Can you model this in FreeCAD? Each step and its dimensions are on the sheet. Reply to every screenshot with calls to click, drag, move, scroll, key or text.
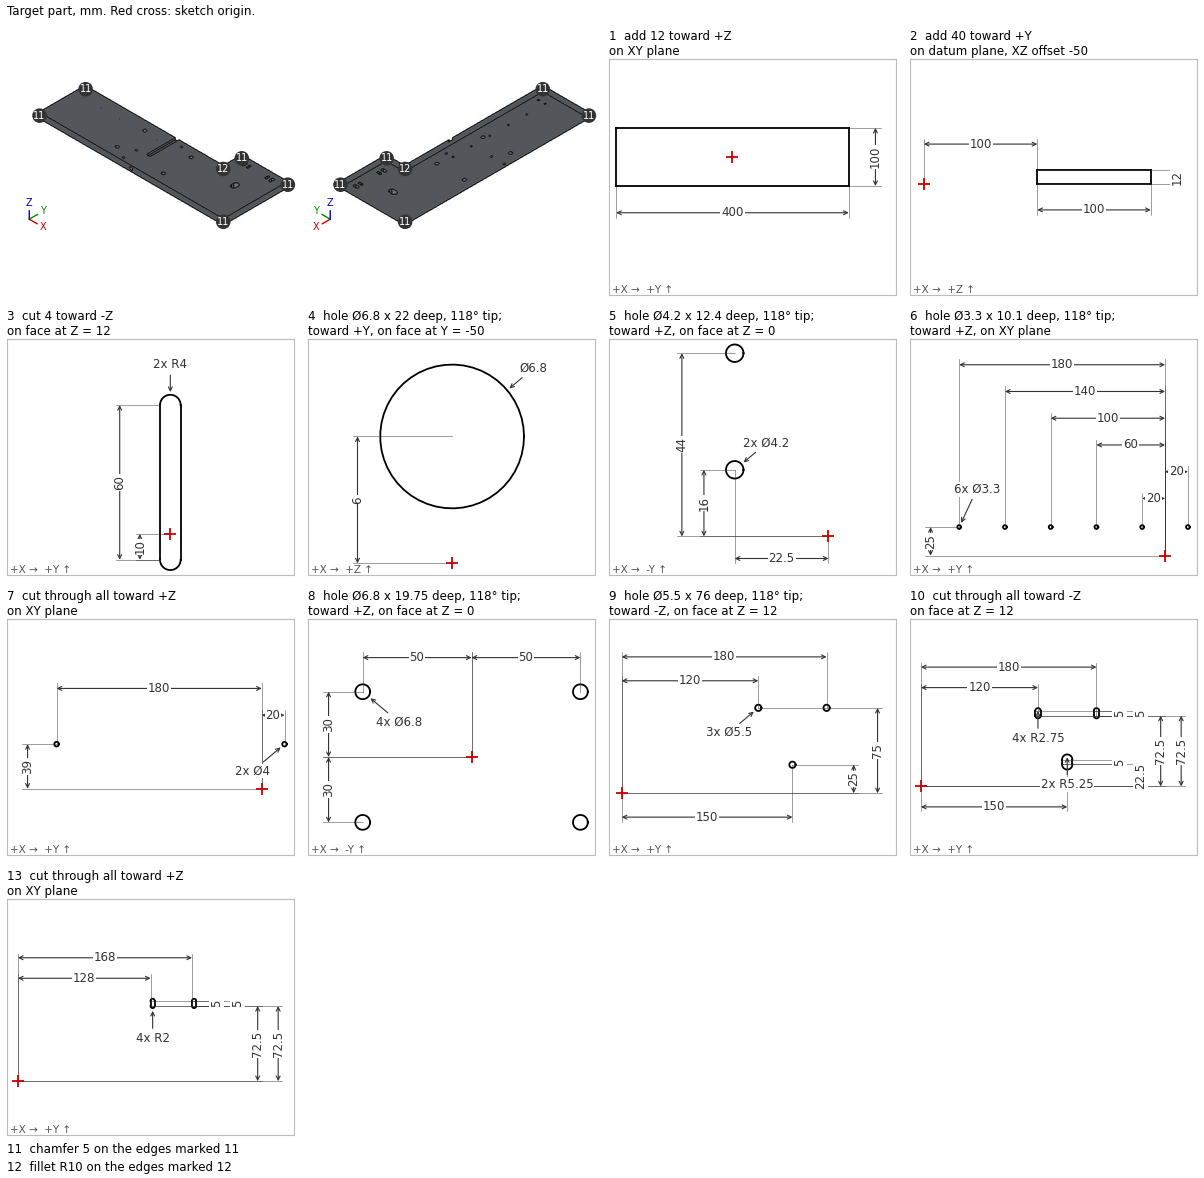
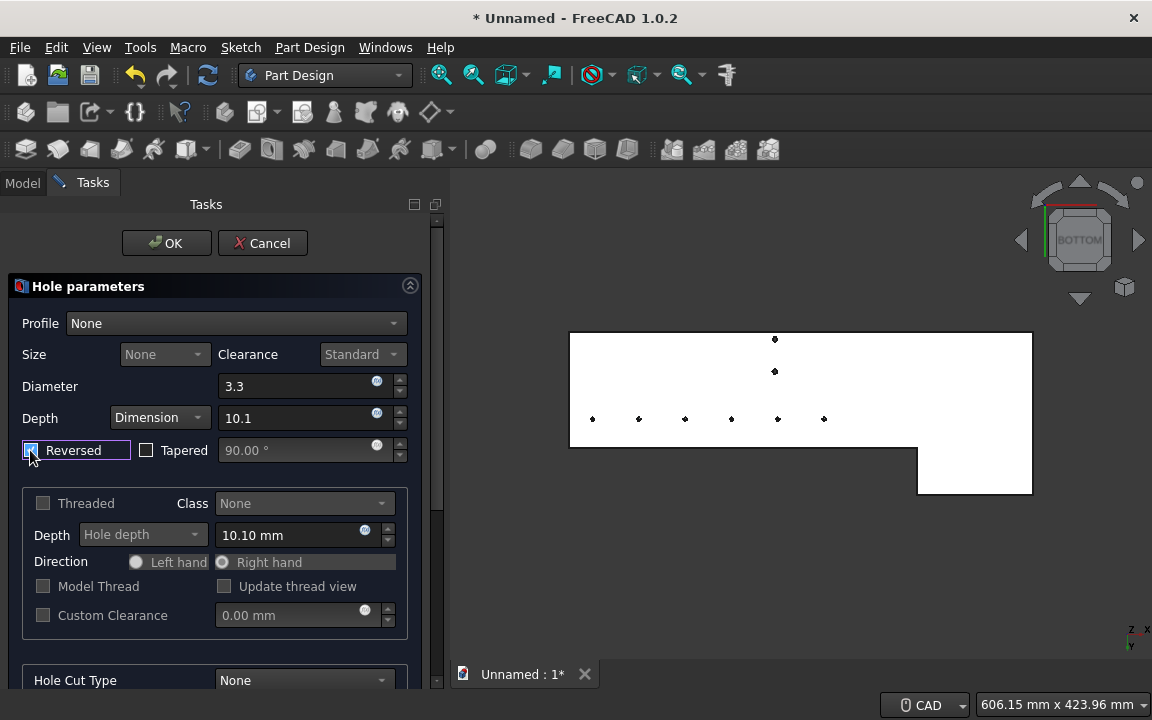
click(167, 243)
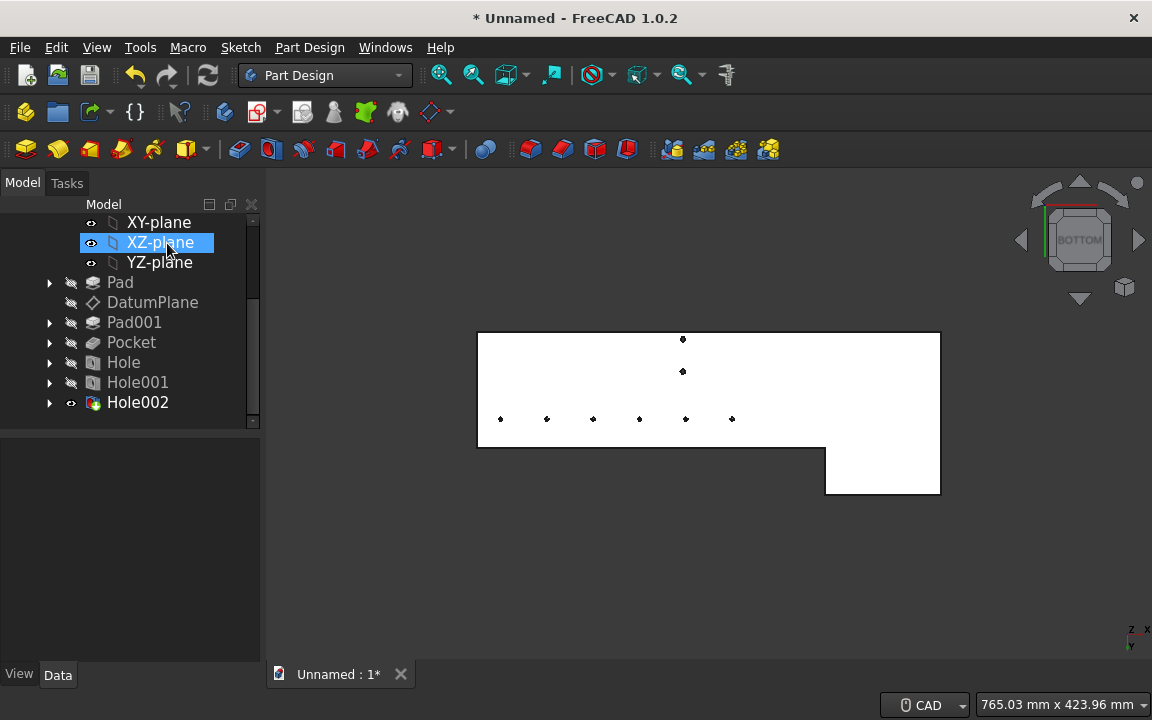
click(258, 112)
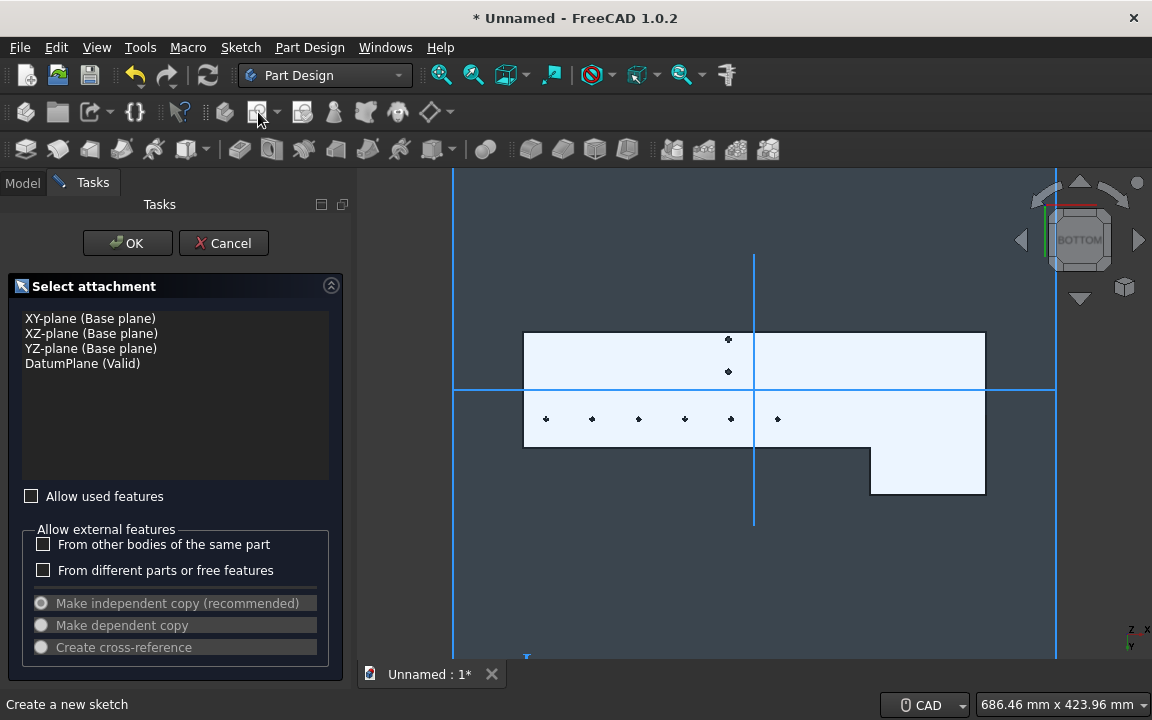
click(82, 318)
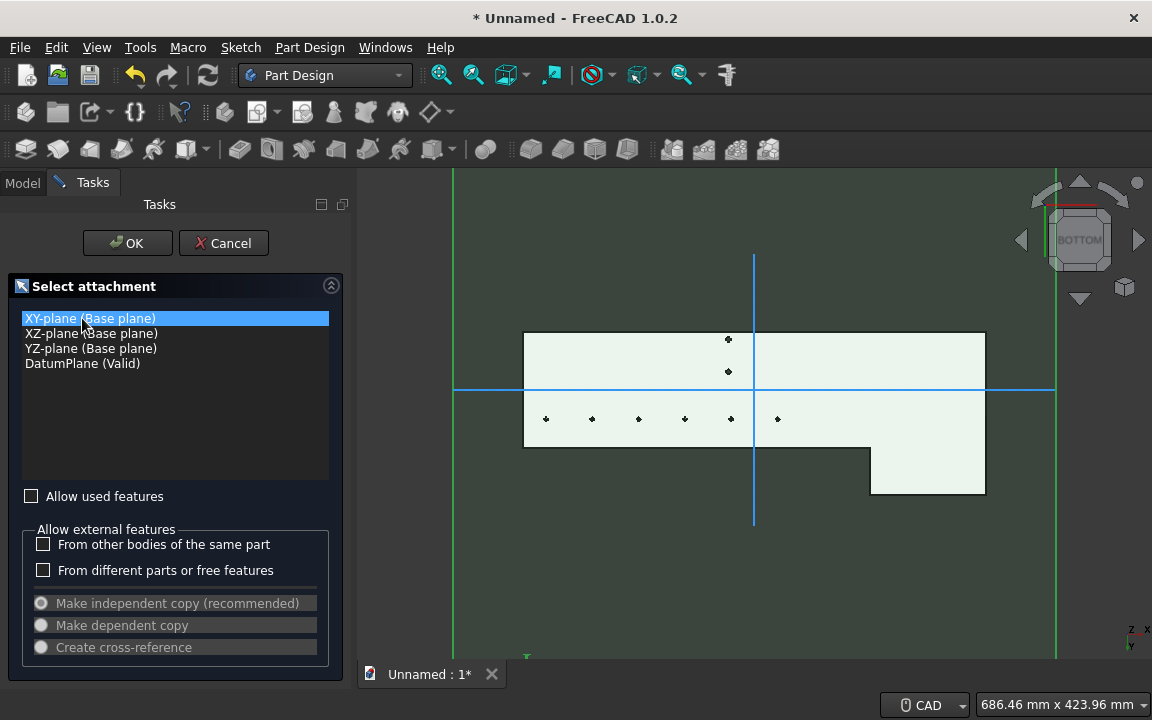
click(128, 243)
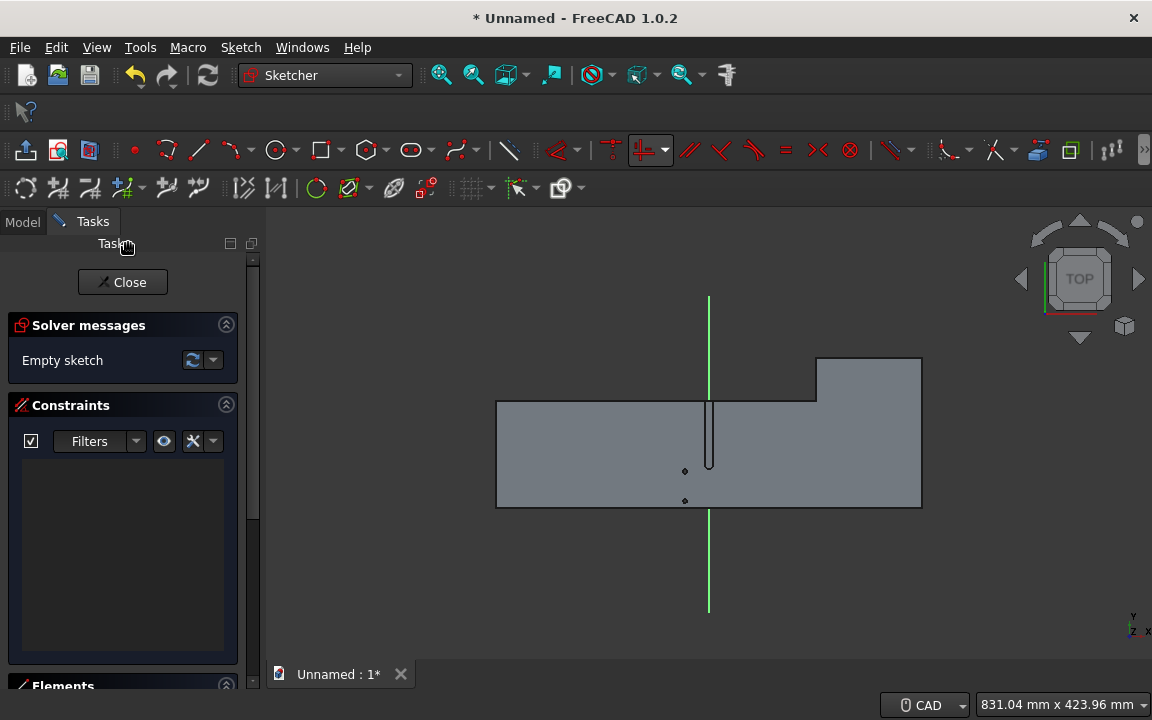
click(90, 150)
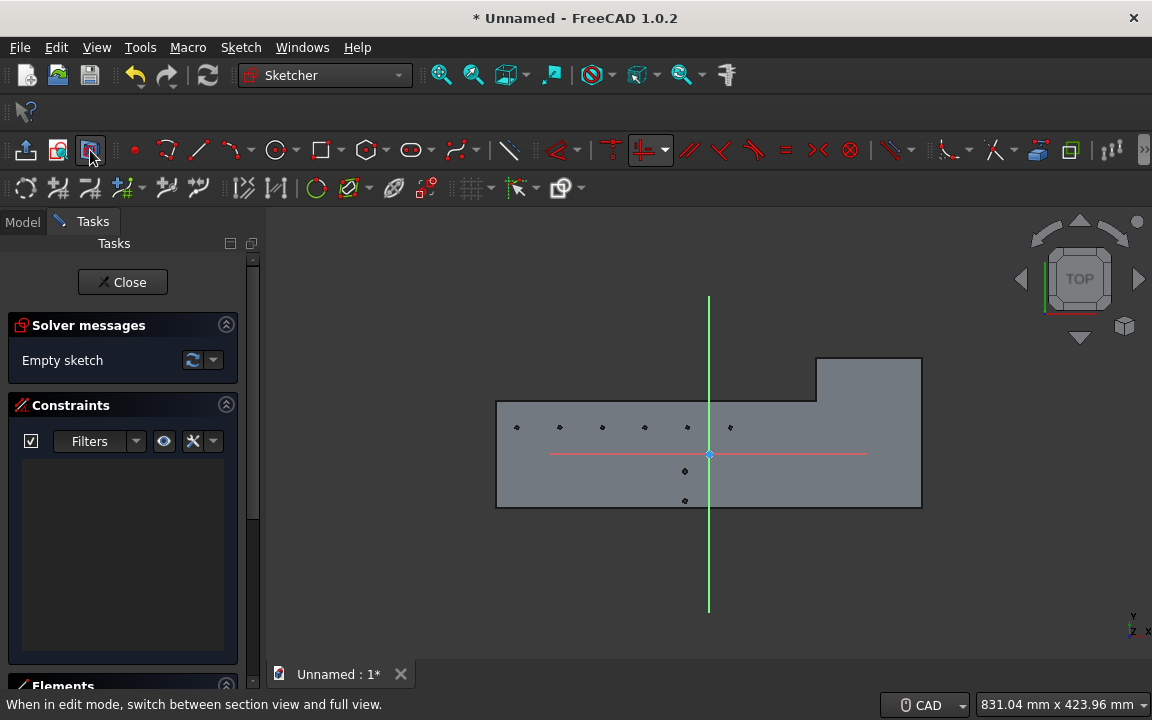
scroll(610, 432, up, 4)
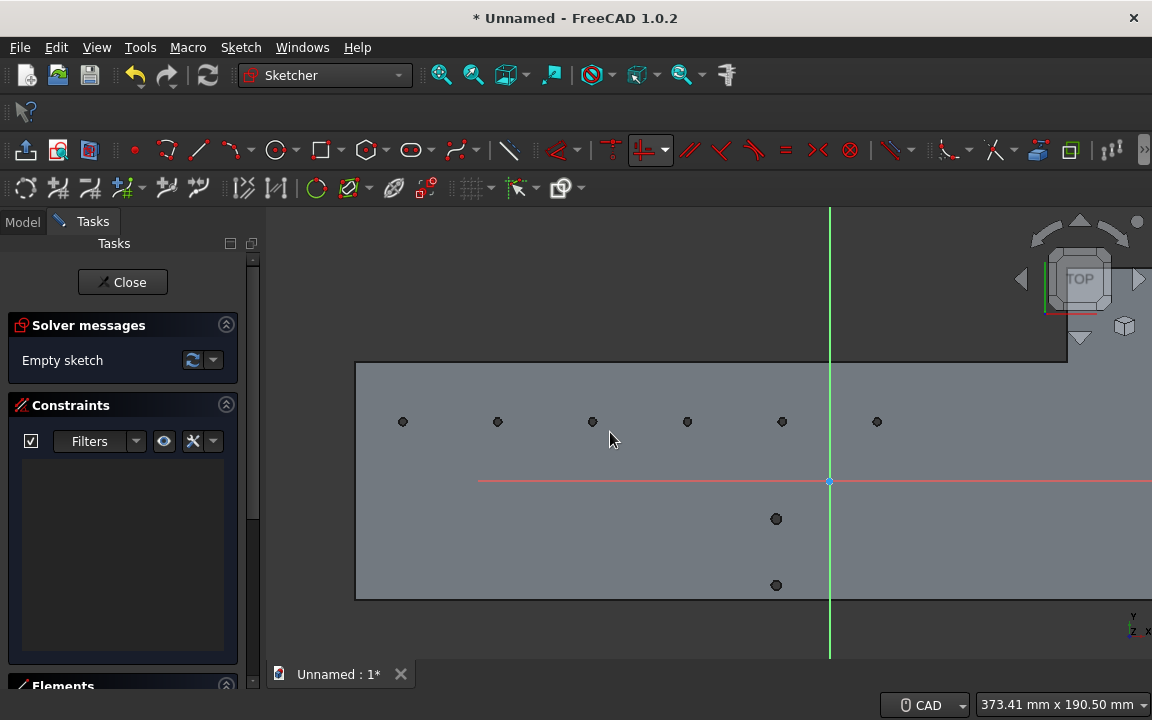
click(276, 150)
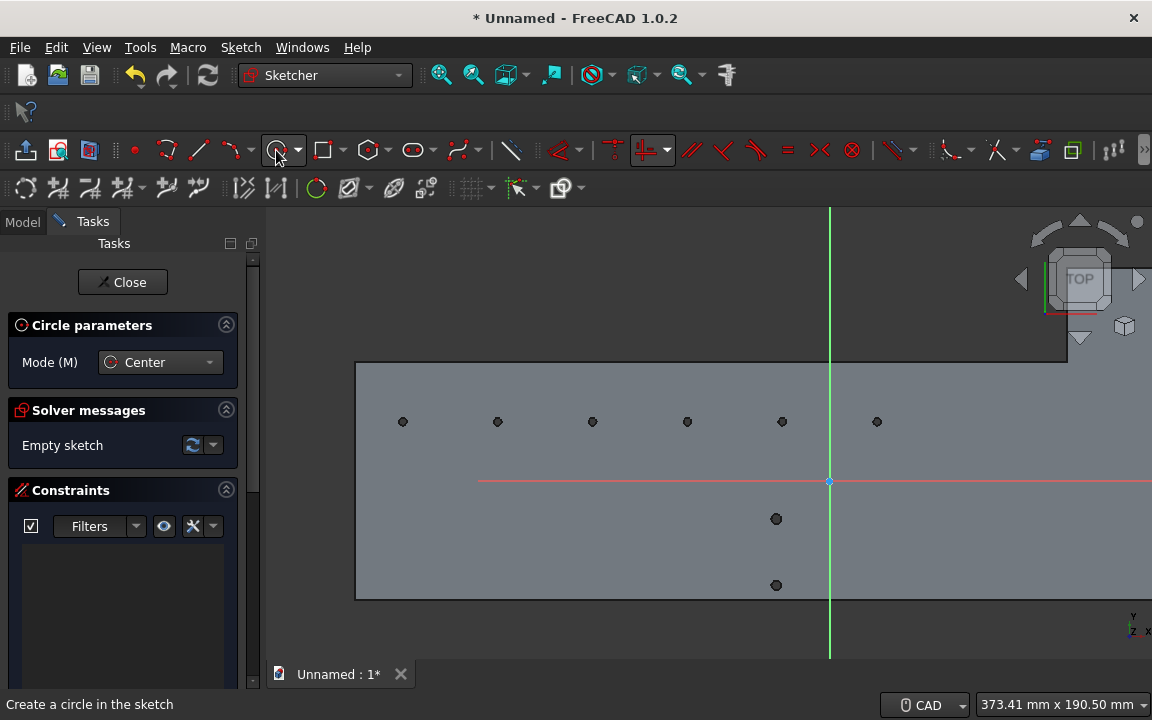
scroll(403, 389, up, 8)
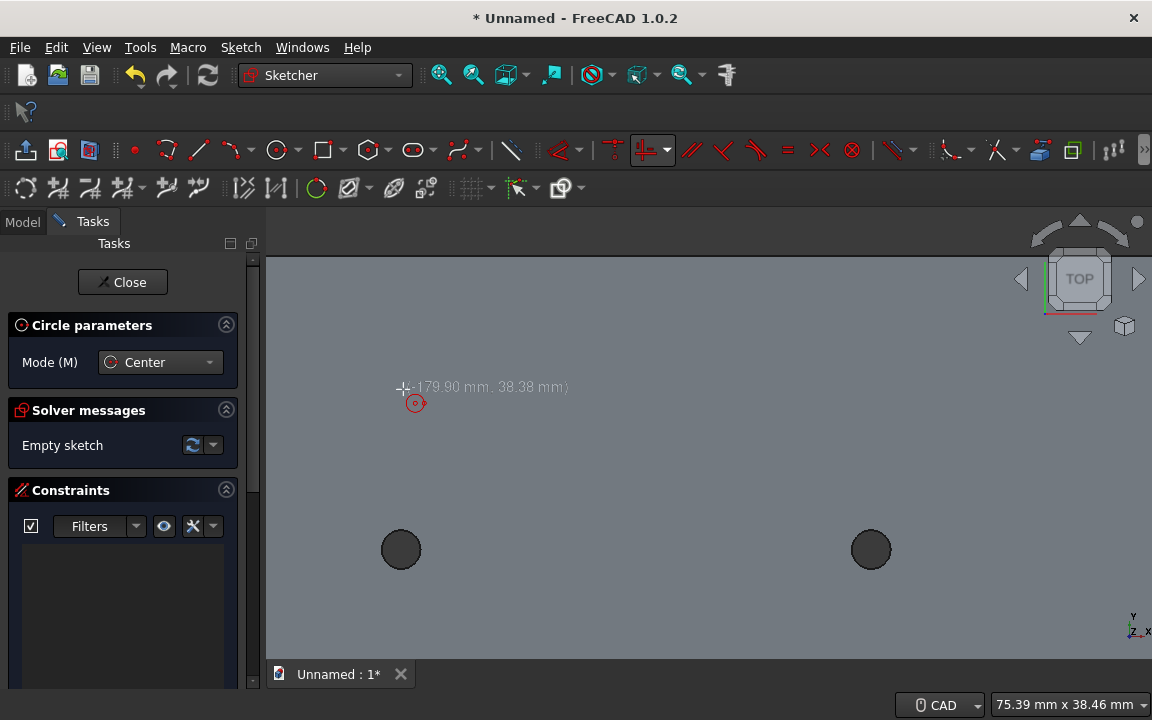
scroll(404, 390, down, 8)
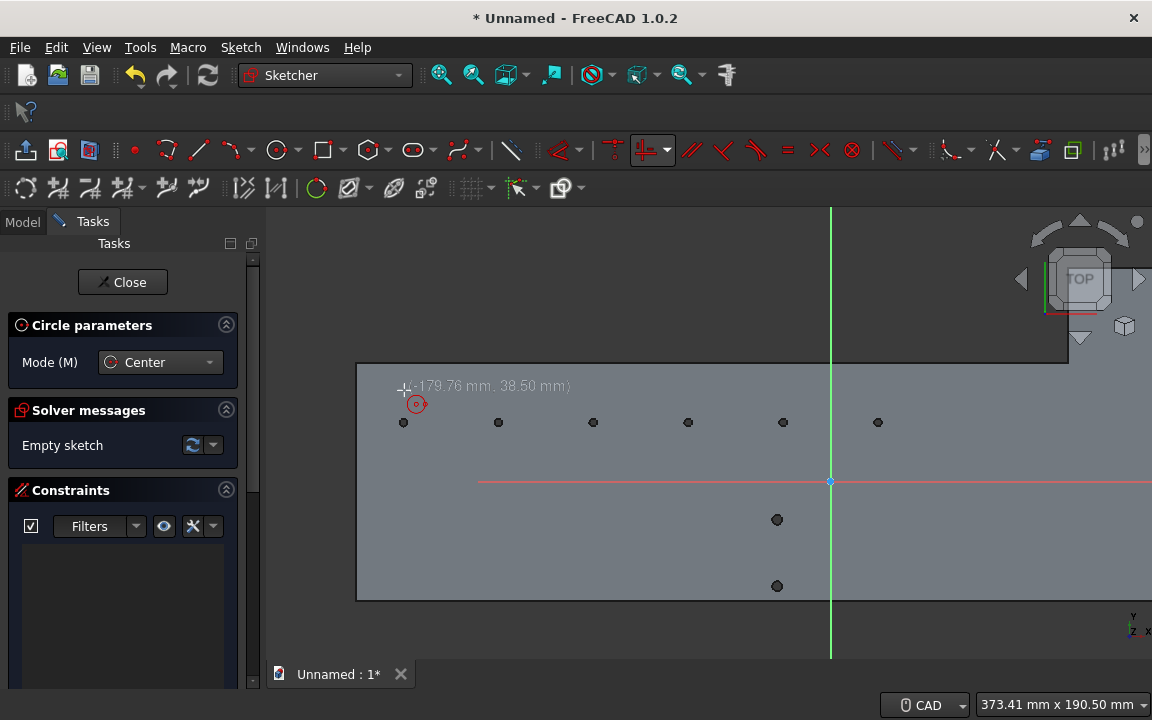
click(404, 389)
move(407, 386)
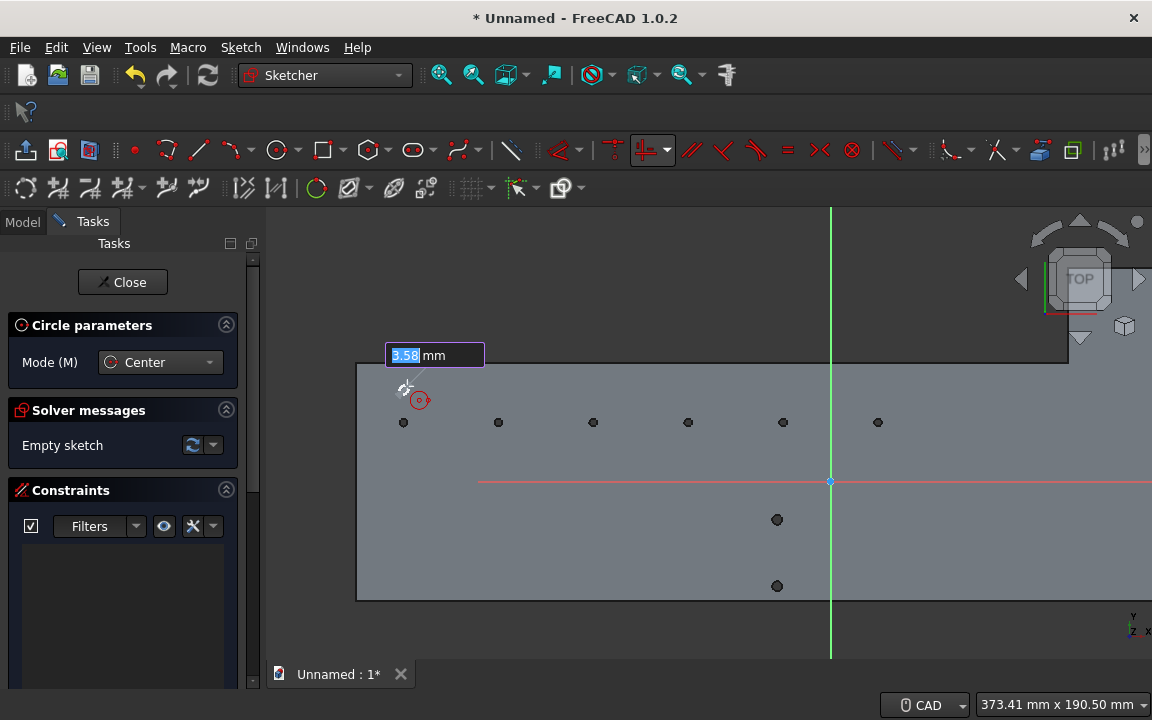
text(4)
key(Return)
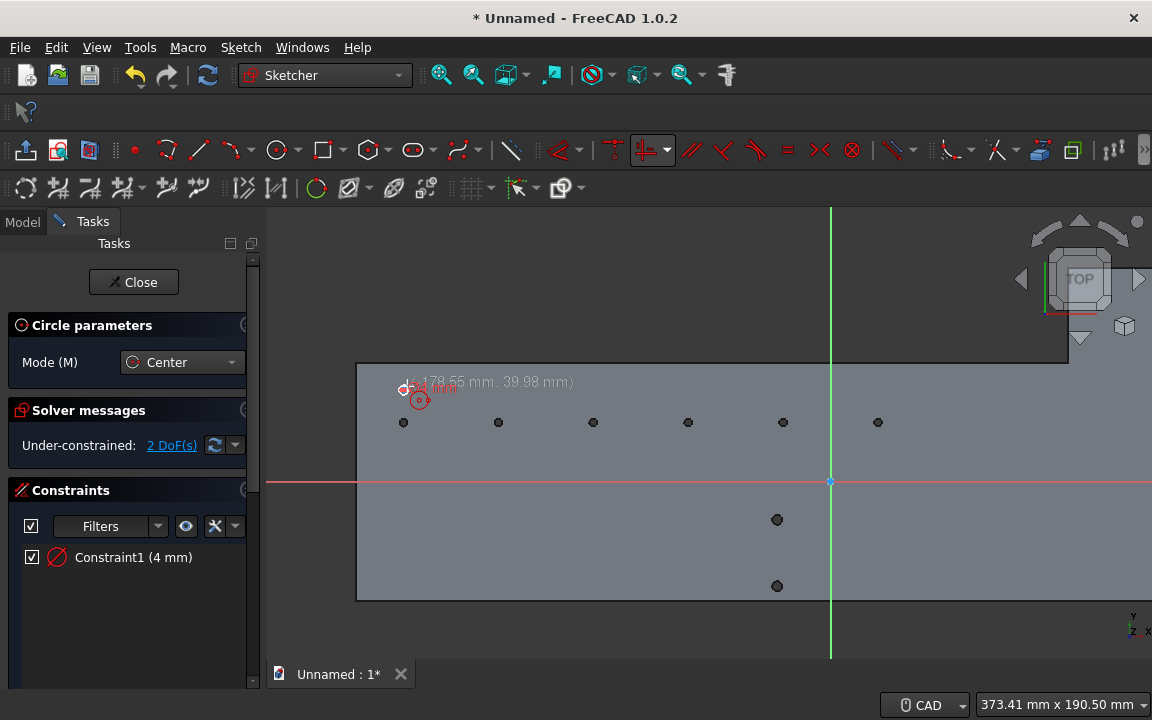
scroll(878, 389, up, 8)